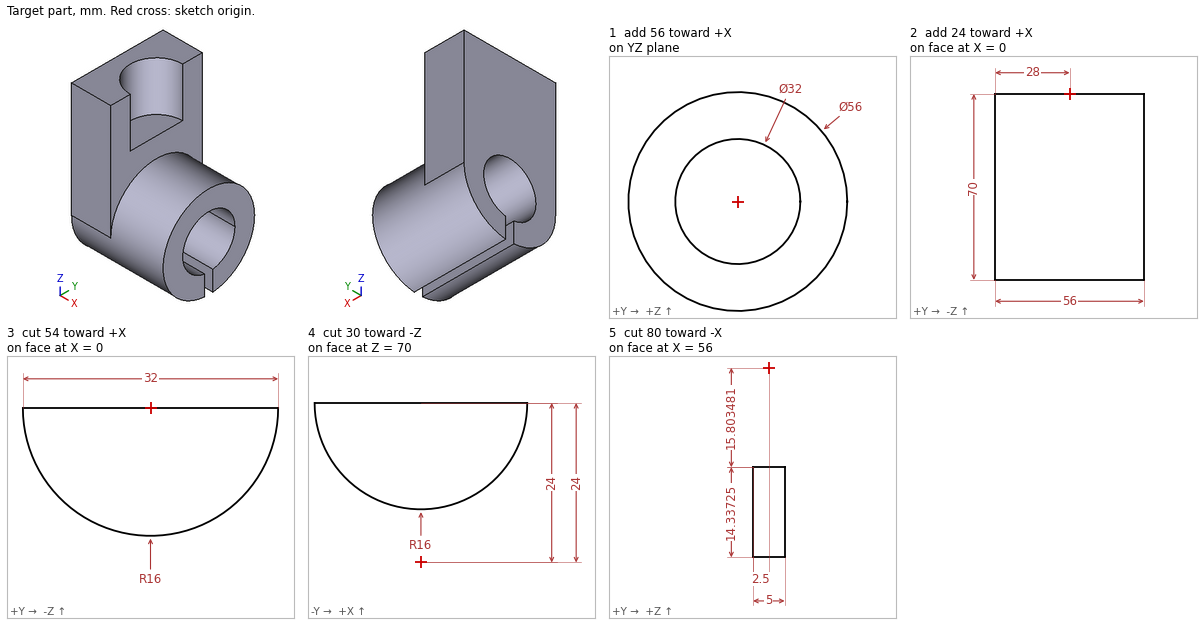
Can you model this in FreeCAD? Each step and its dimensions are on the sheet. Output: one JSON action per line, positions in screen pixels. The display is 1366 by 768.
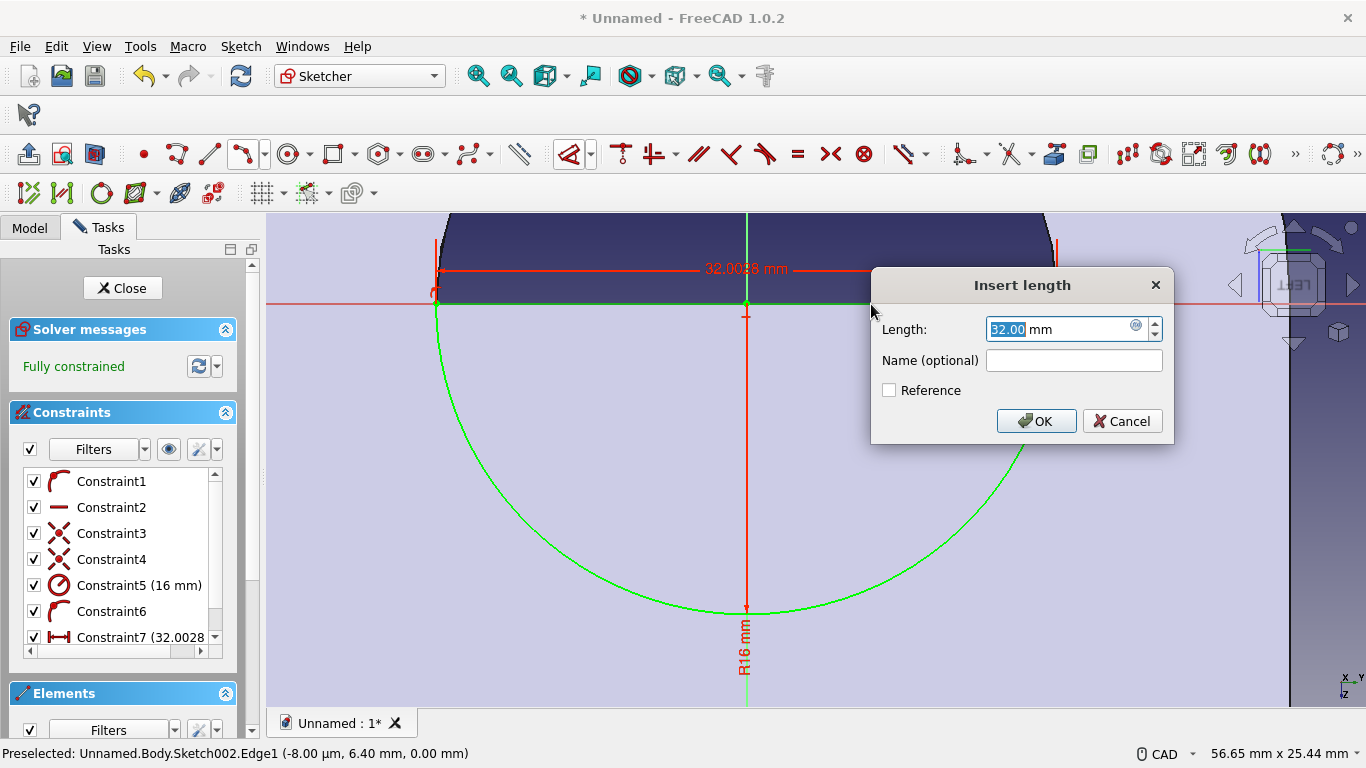
{"action": "type", "text": "32"}
{"action": "key", "text": "Return"}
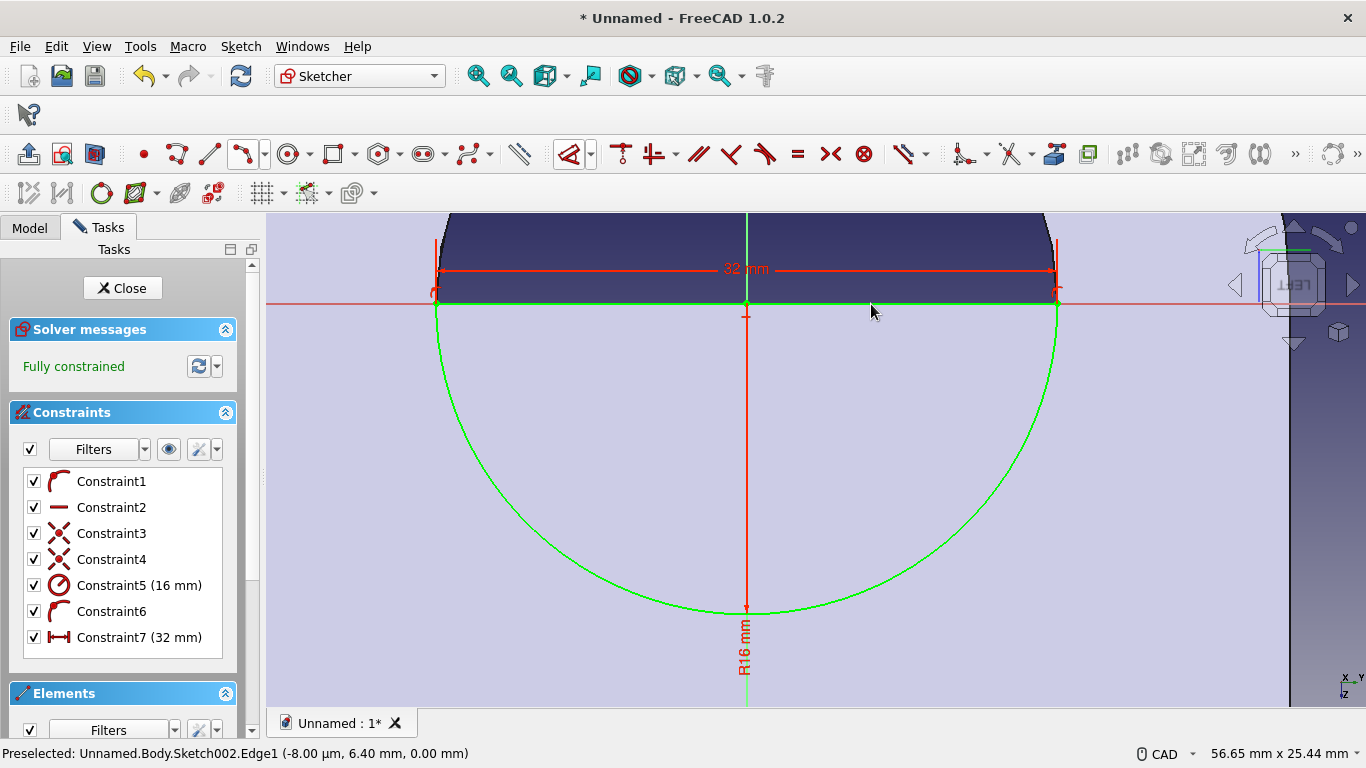
{"action": "left_click", "coordinate": [123, 288]}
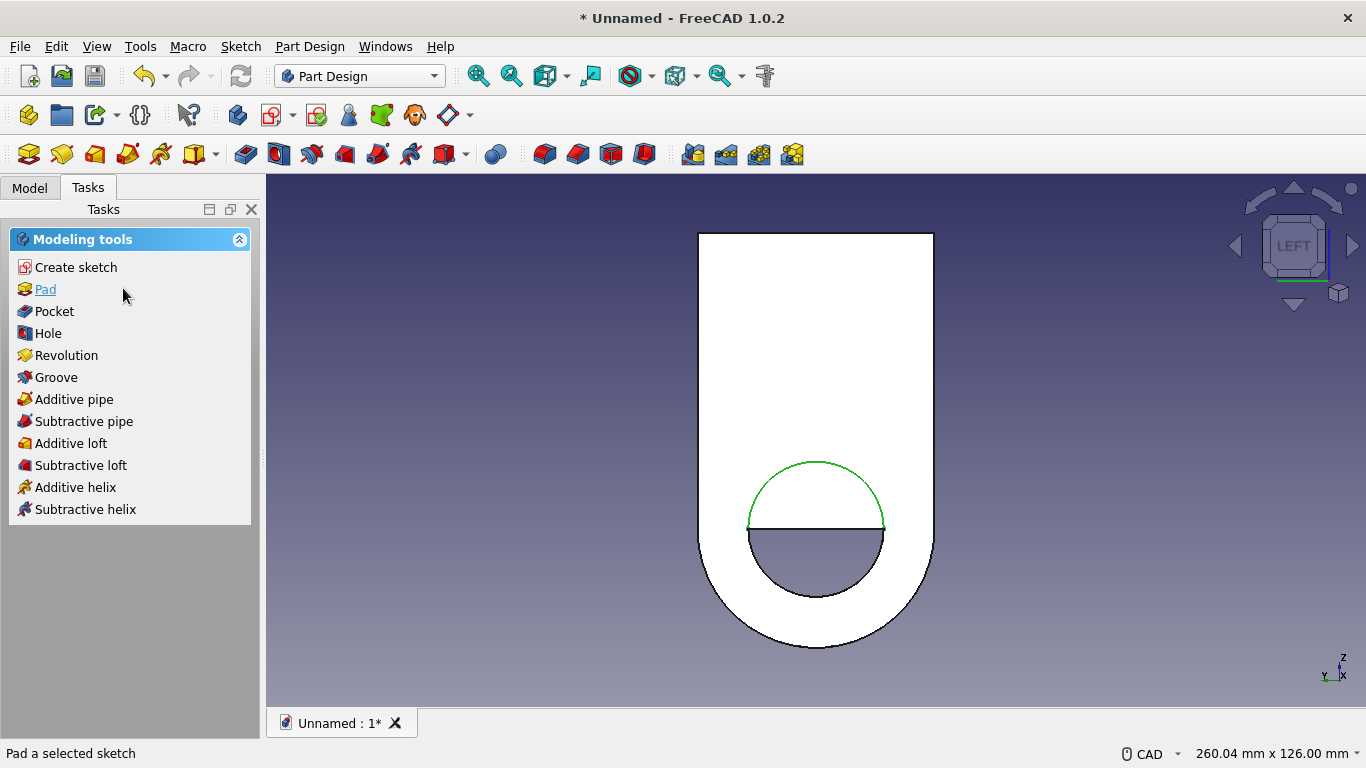
{"action": "left_click", "coordinate": [246, 154]}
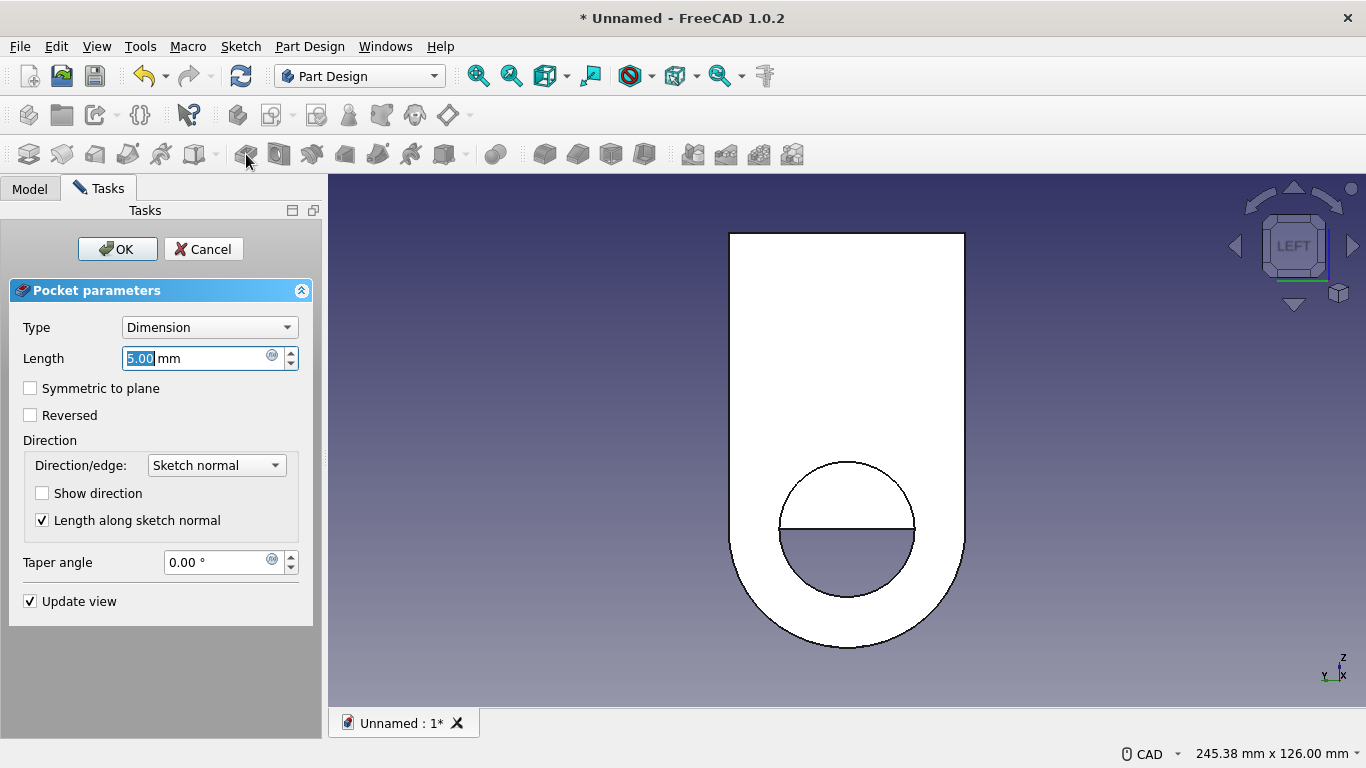
{"action": "type", "text": "54"}
{"action": "key", "text": "Tab"}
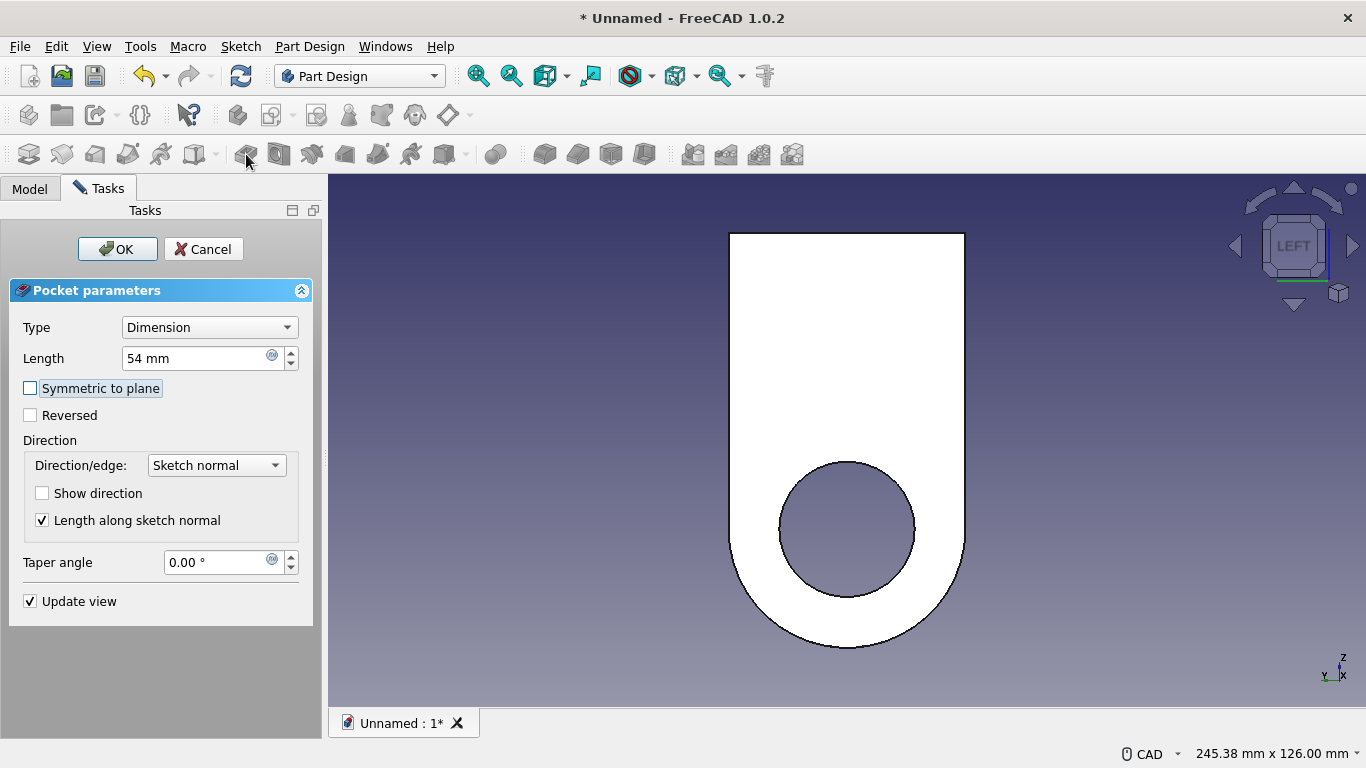
{"action": "left_click", "coordinate": [118, 249]}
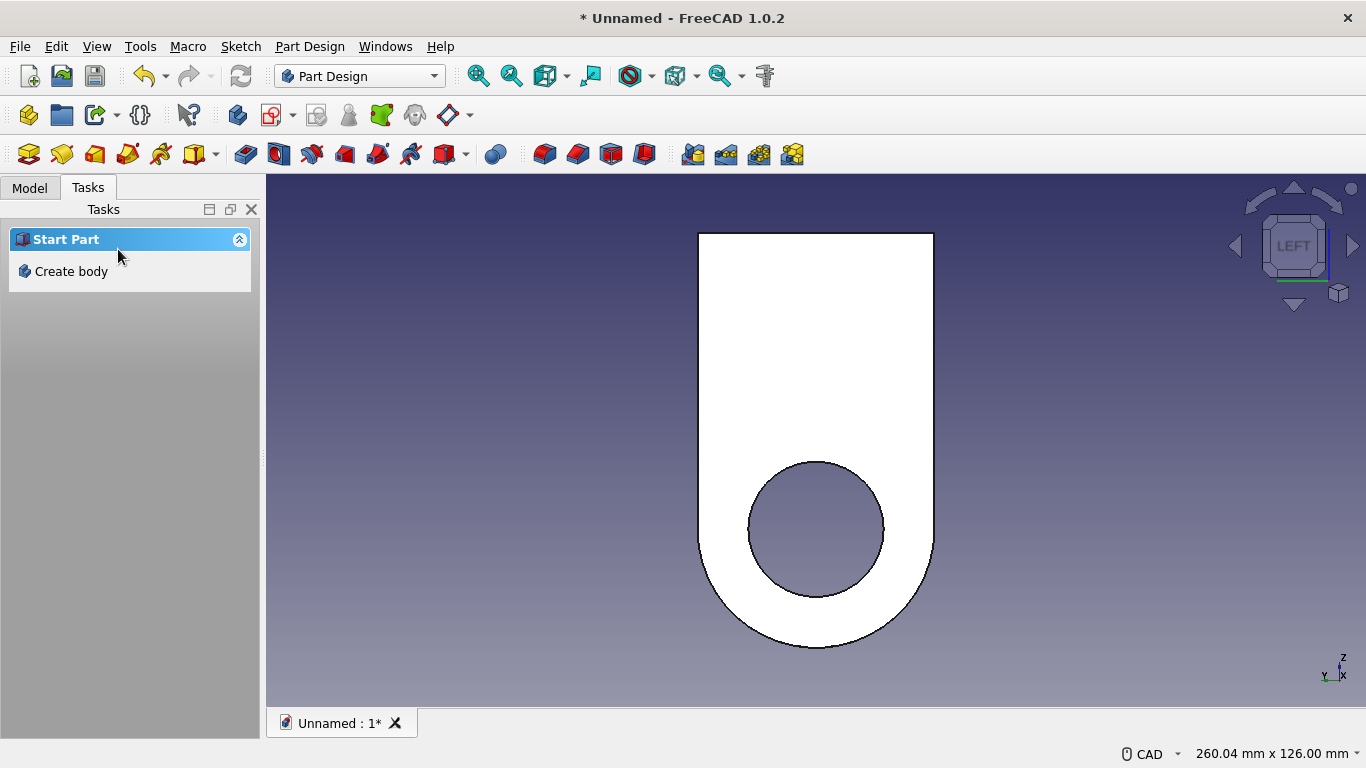
{"action": "key", "text": "0"}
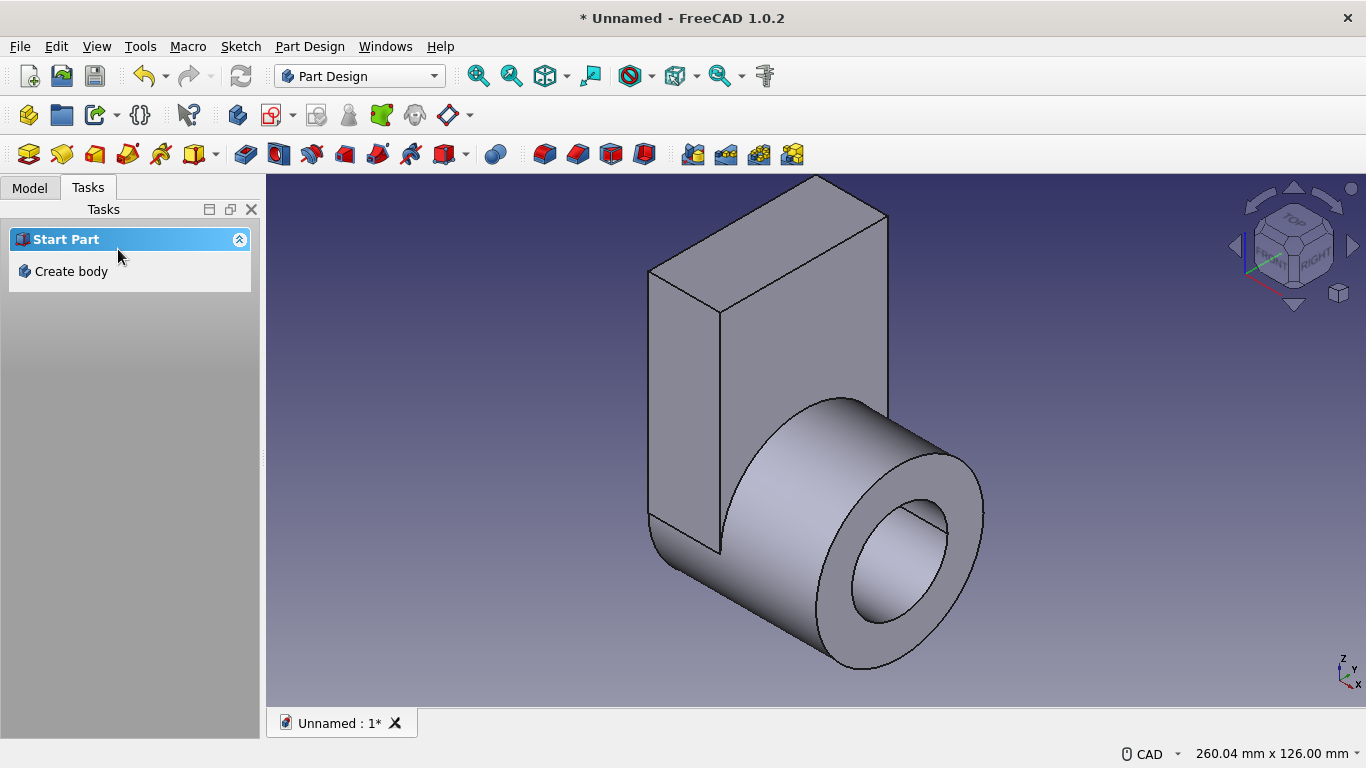
{"action": "left_click", "coordinate": [816, 215]}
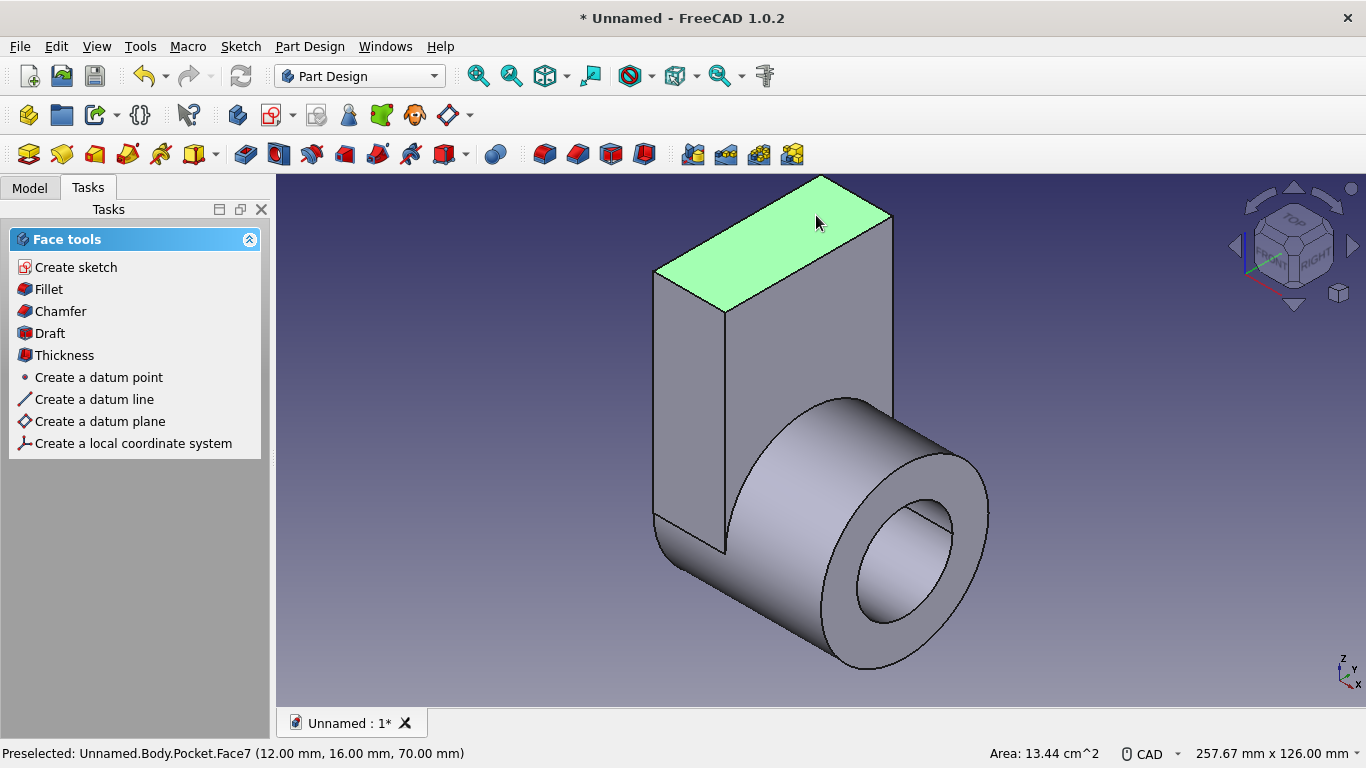
{"action": "left_click", "coordinate": [270, 116]}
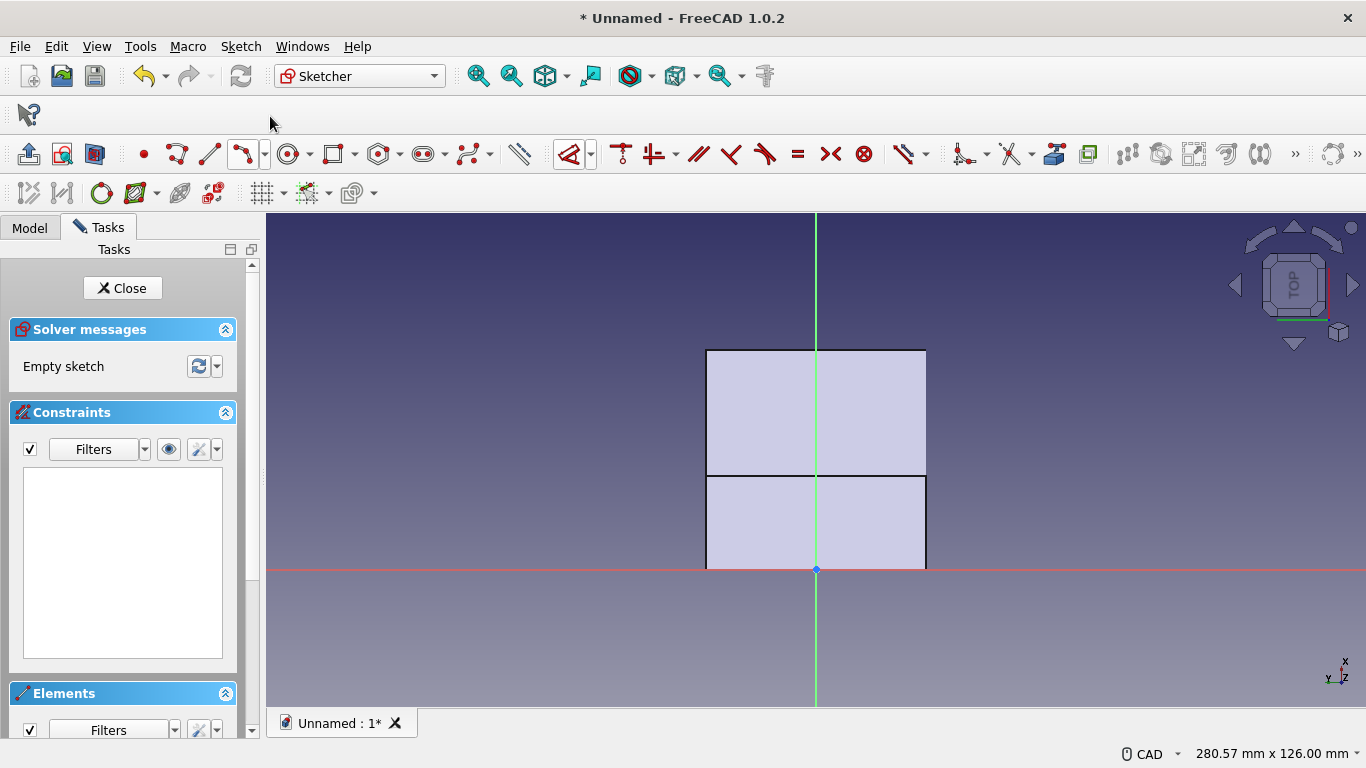
{"action": "scroll", "coordinate": [846, 550], "scroll_direction": "up", "scroll_amount": 6}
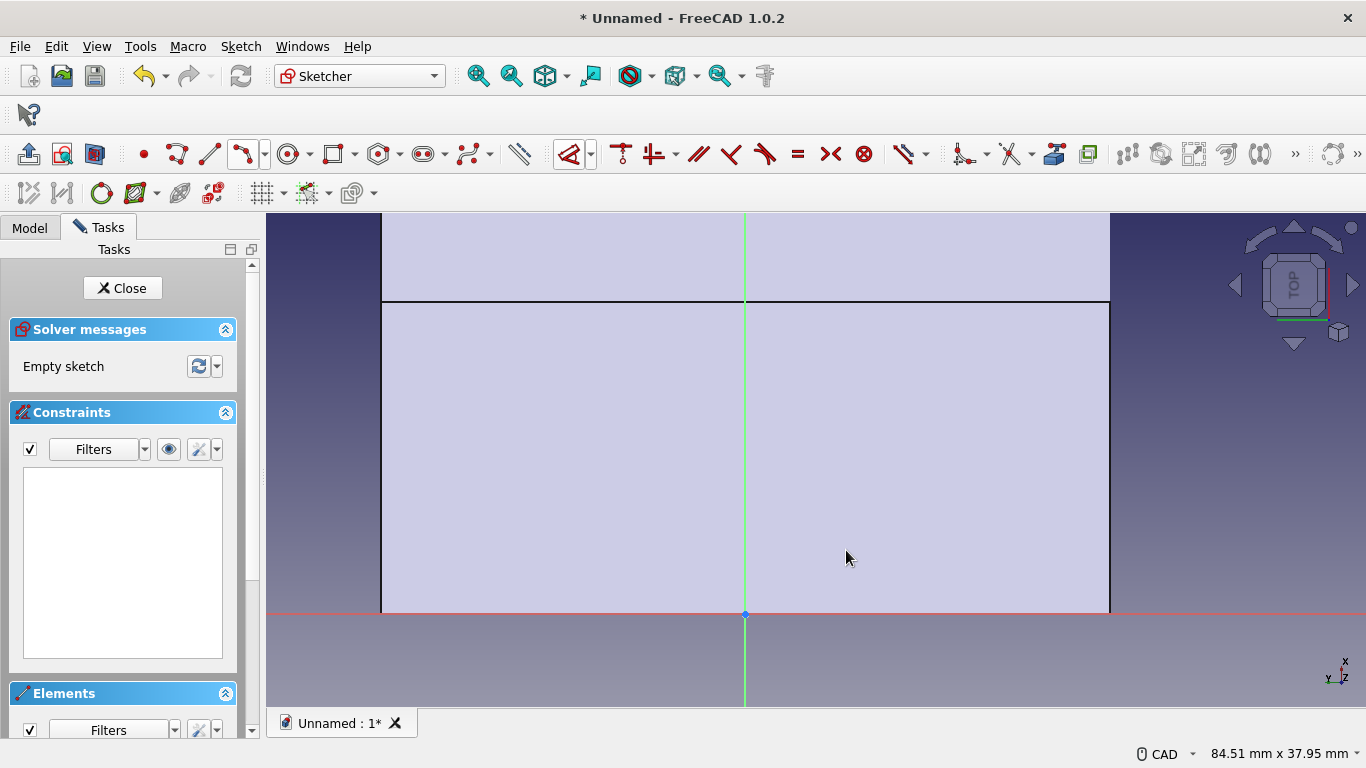
{"action": "left_click", "coordinate": [210, 154]}